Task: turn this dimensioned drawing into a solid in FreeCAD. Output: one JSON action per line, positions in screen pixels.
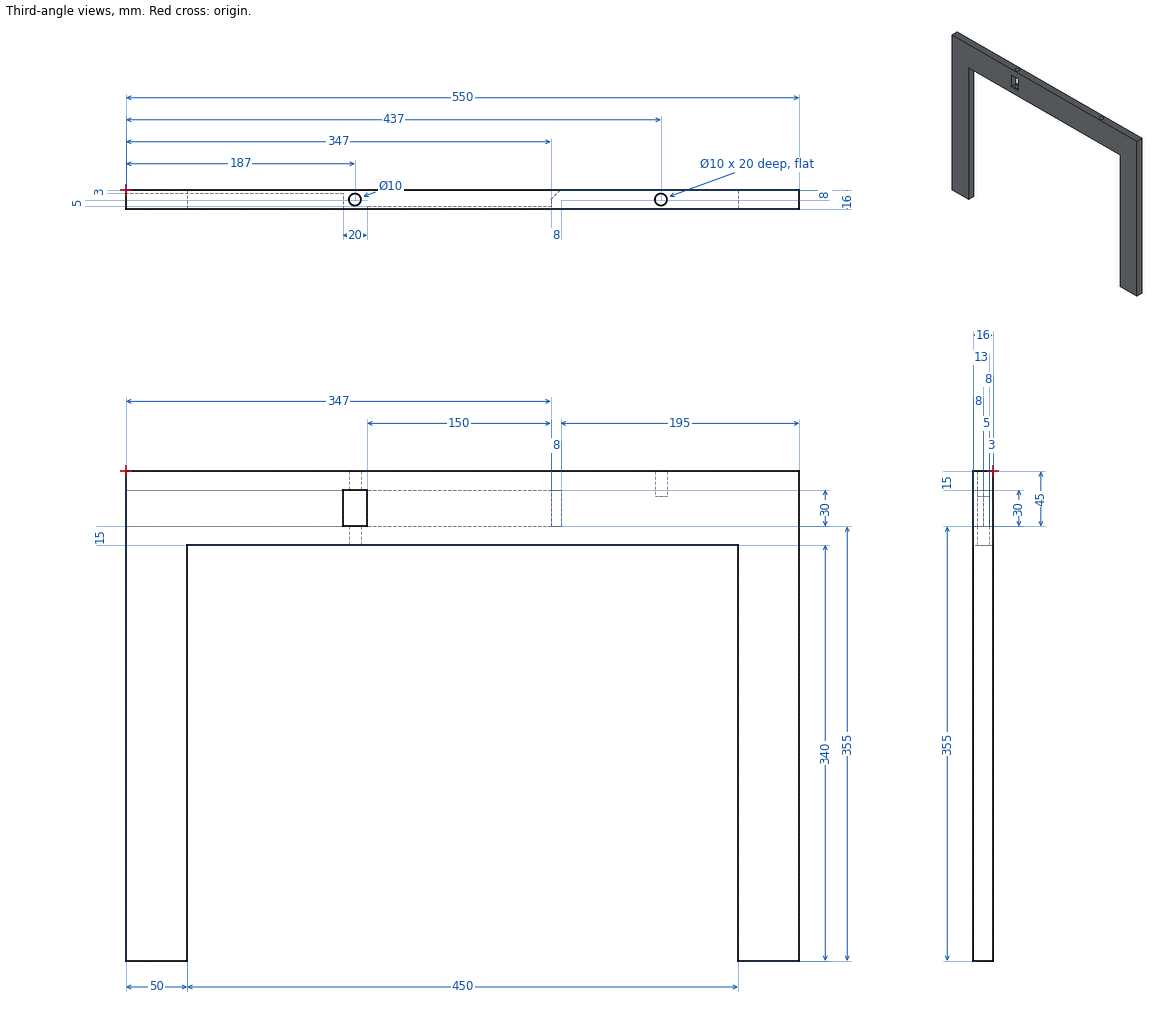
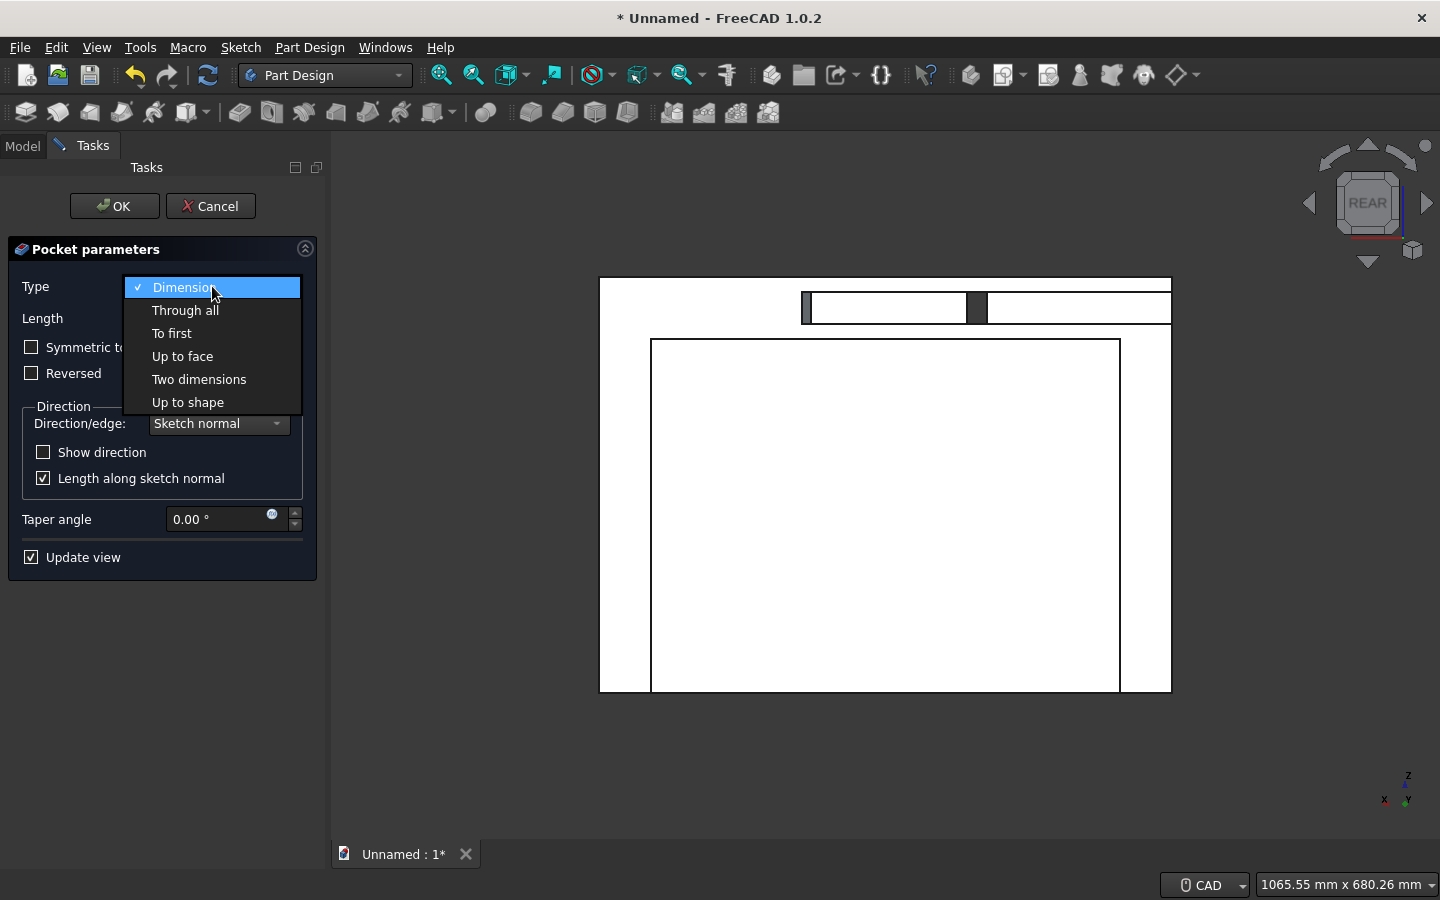
{"action": "left_click", "coordinate": [212, 310]}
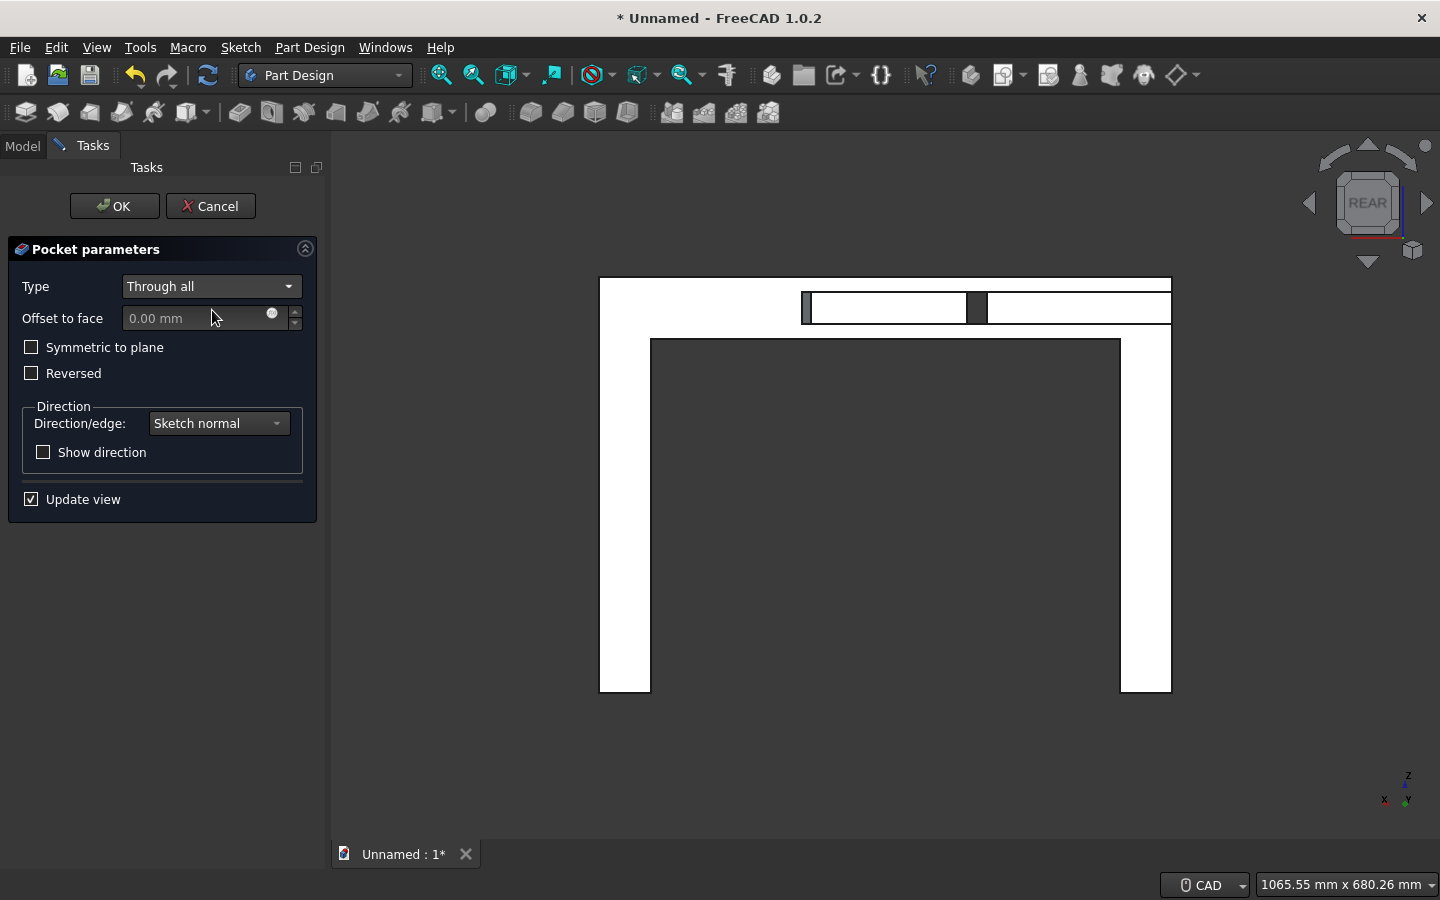
{"action": "left_click", "coordinate": [115, 206]}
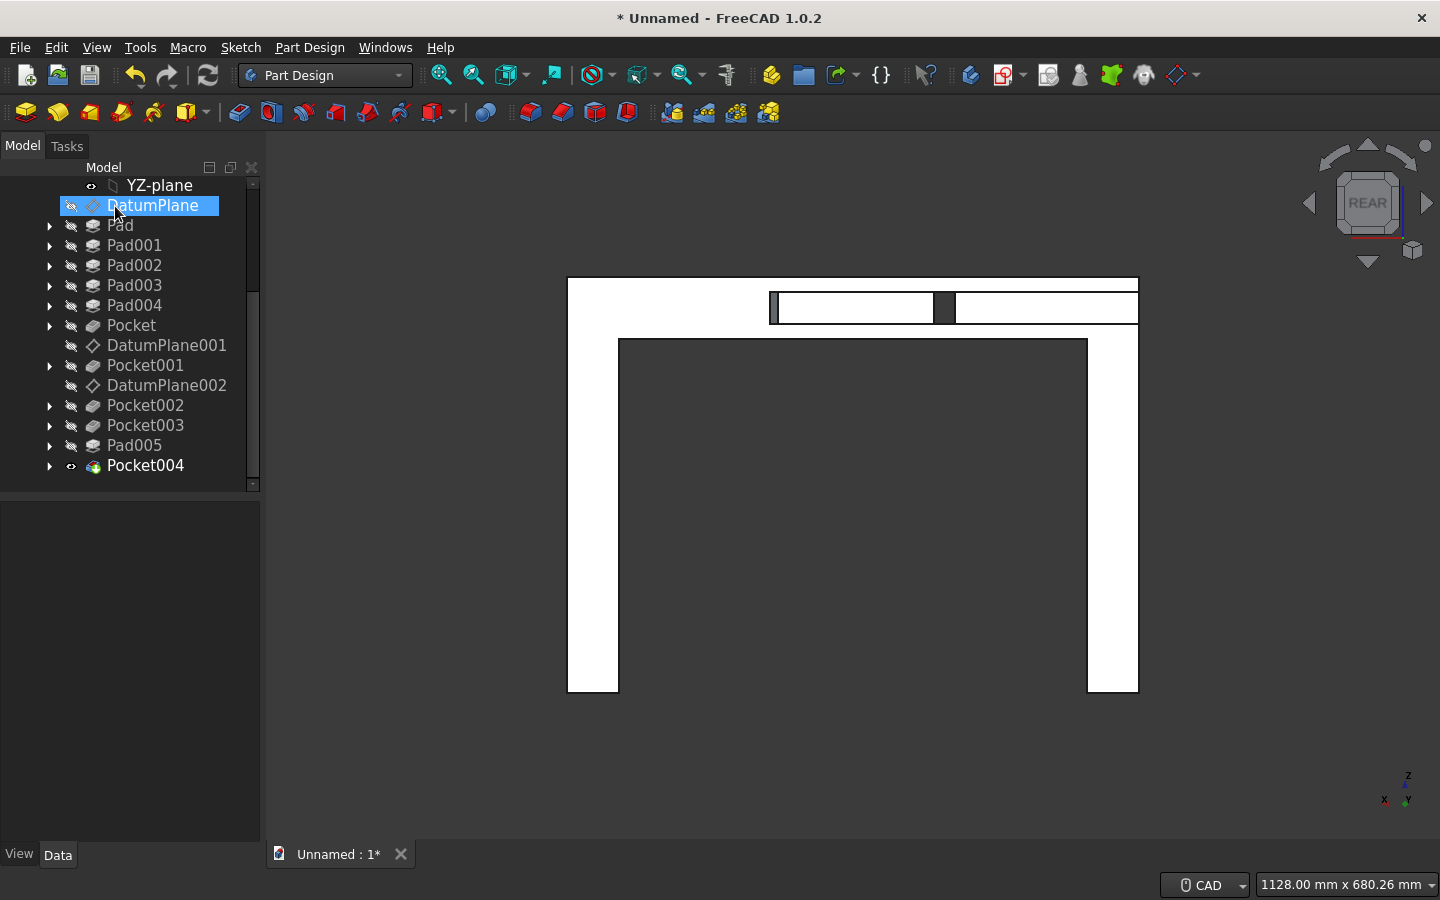
{"action": "key", "text": "0"}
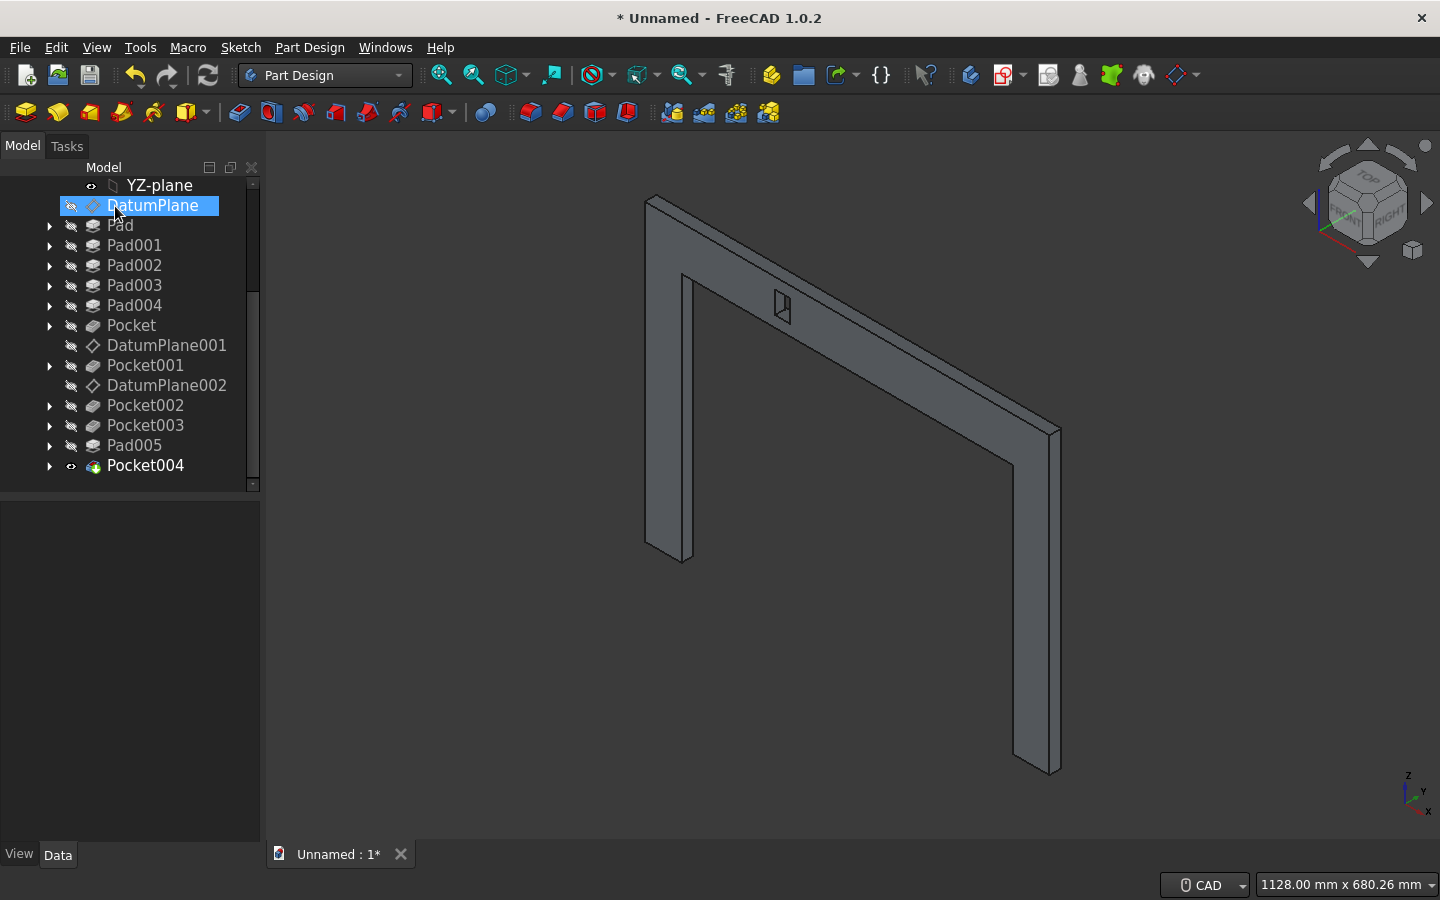
{"action": "key", "text": "2"}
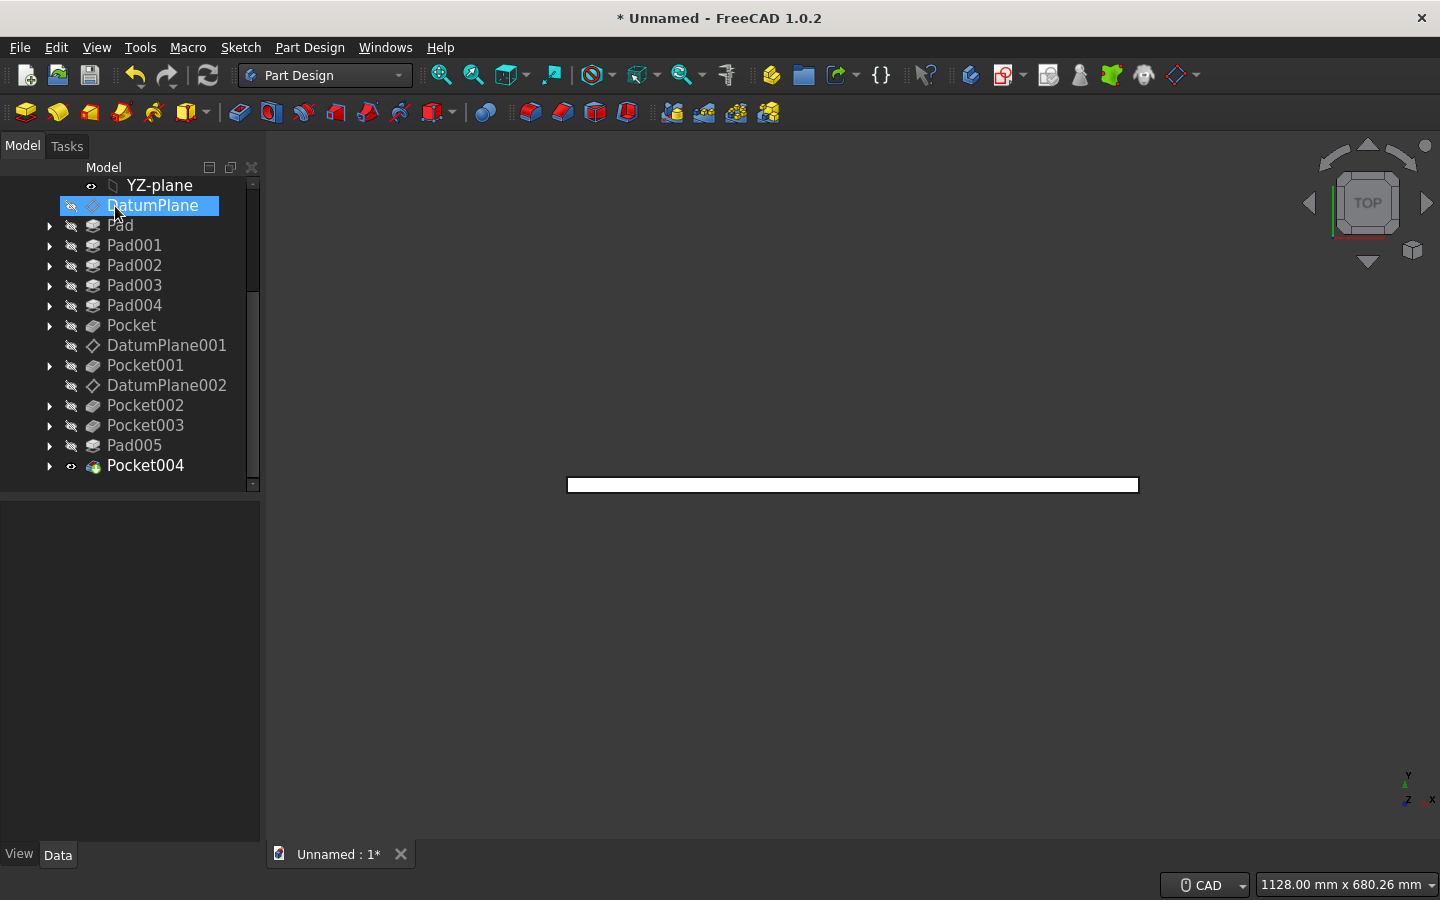
{"action": "left_click", "coordinate": [1098, 484]}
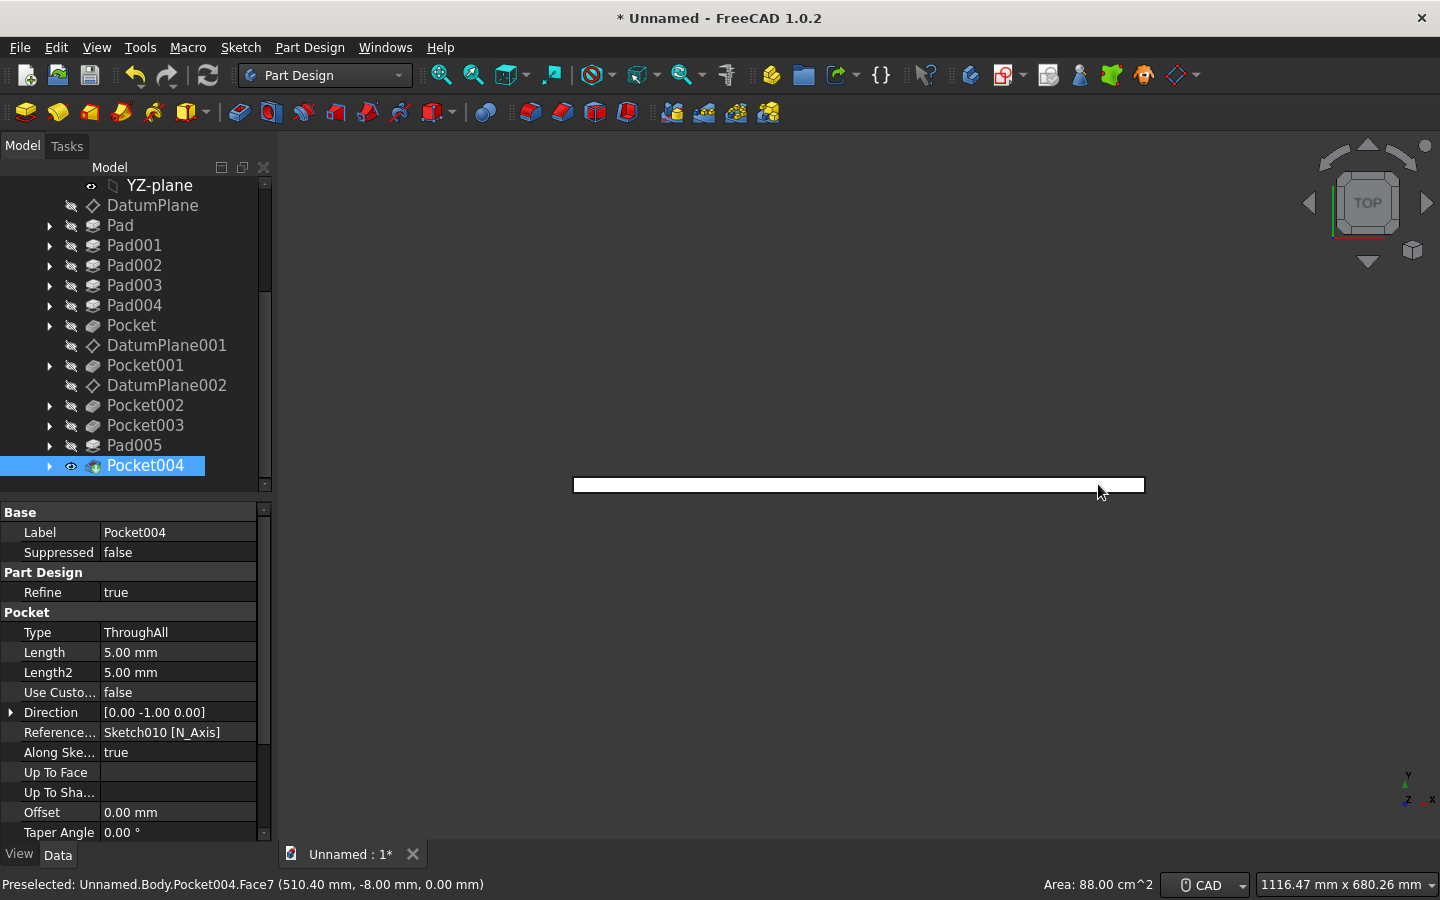
{"action": "left_click", "coordinate": [1004, 76]}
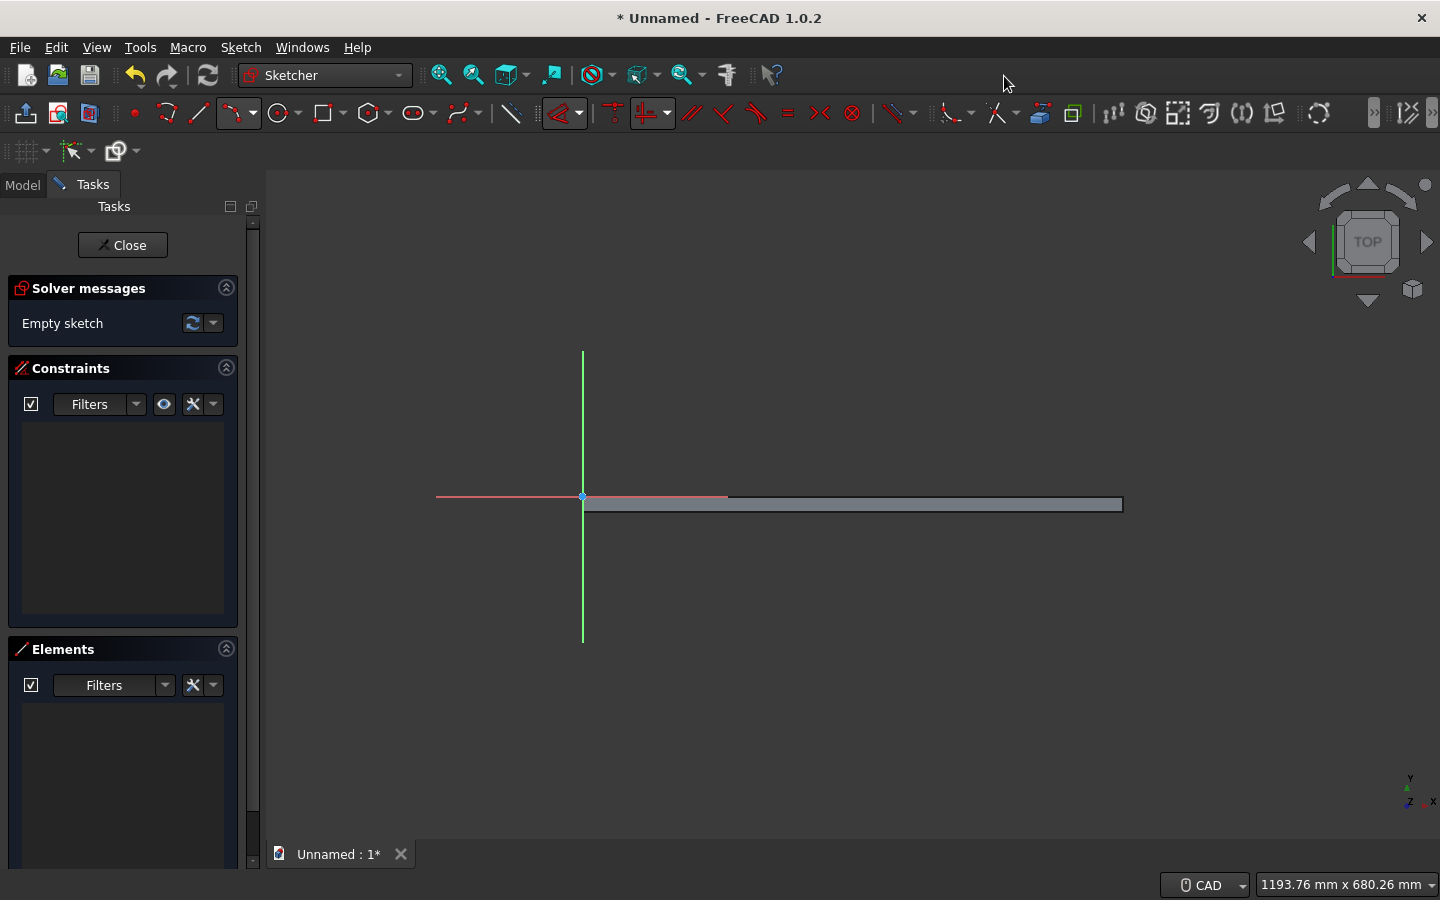
{"action": "scroll", "coordinate": [1024, 504], "scroll_direction": "up", "scroll_amount": 15}